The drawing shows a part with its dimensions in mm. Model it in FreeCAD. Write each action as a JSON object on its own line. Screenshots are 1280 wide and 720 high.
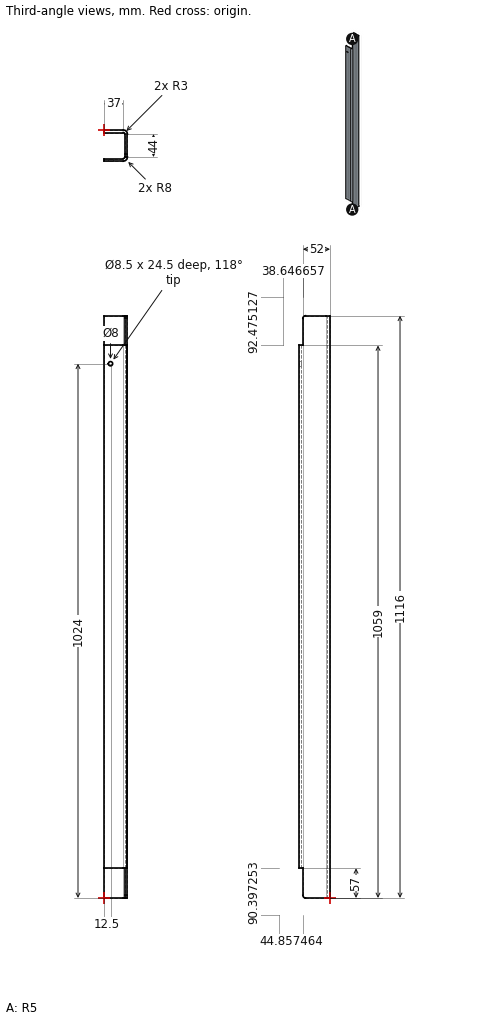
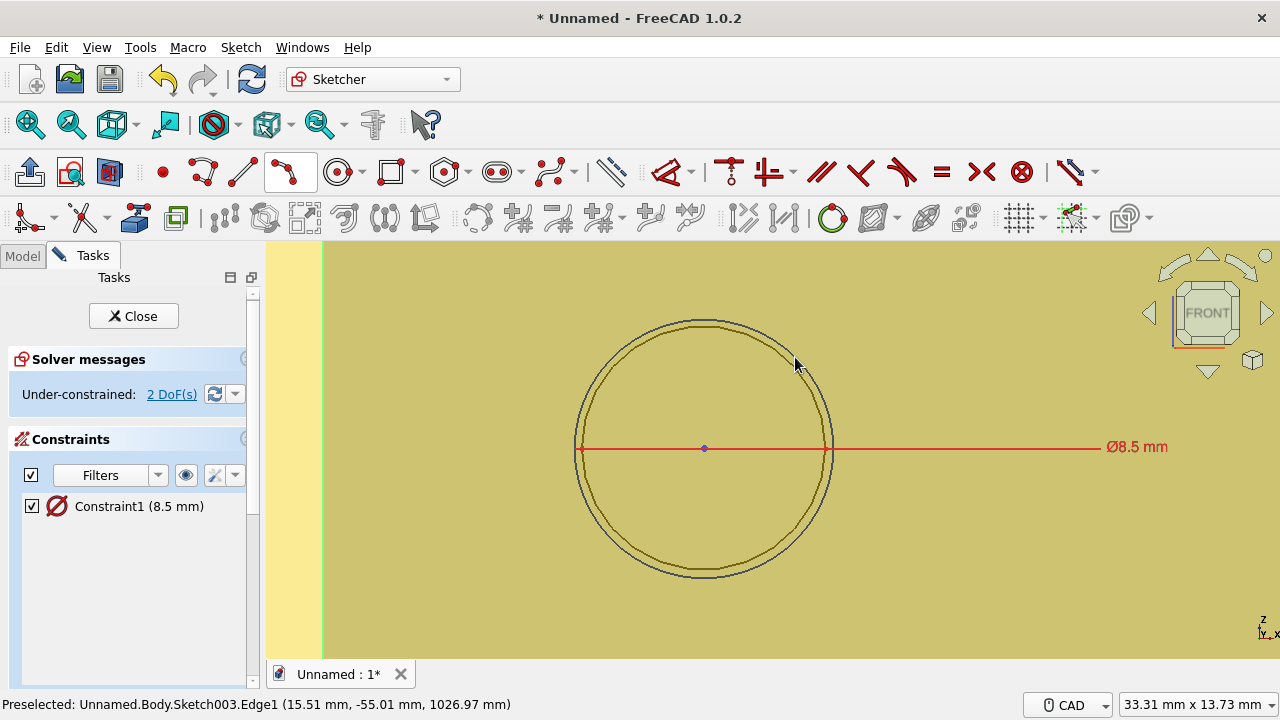
{"action": "key", "text": "d"}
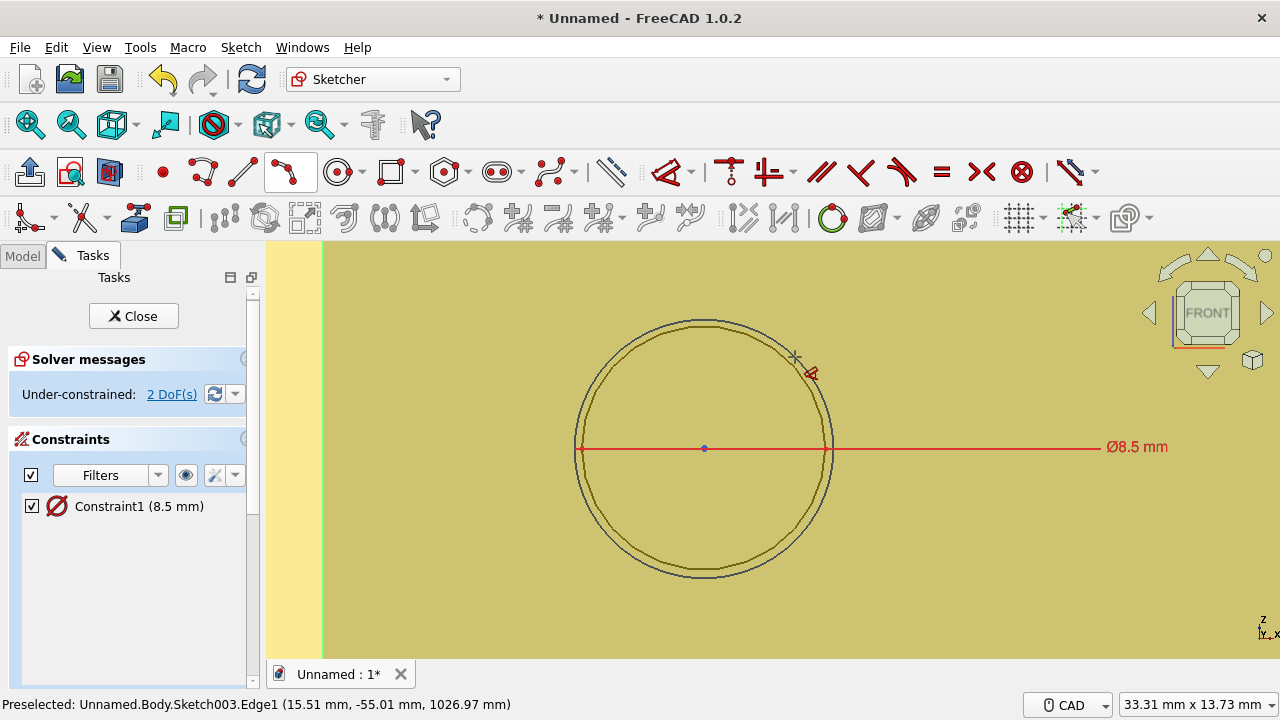
{"action": "left_click", "coordinate": [704, 449]}
{"action": "left_click", "coordinate": [514, 415]}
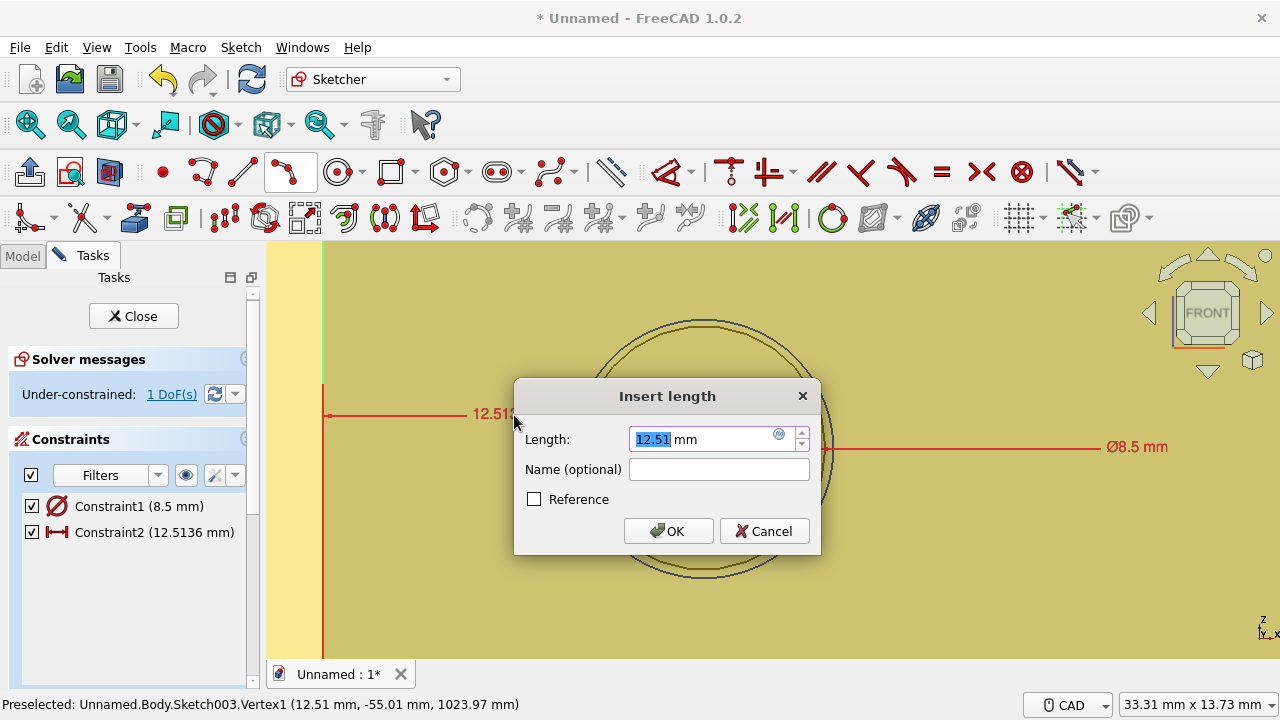
{"action": "type", "text": "12.5"}
{"action": "key", "text": "Return"}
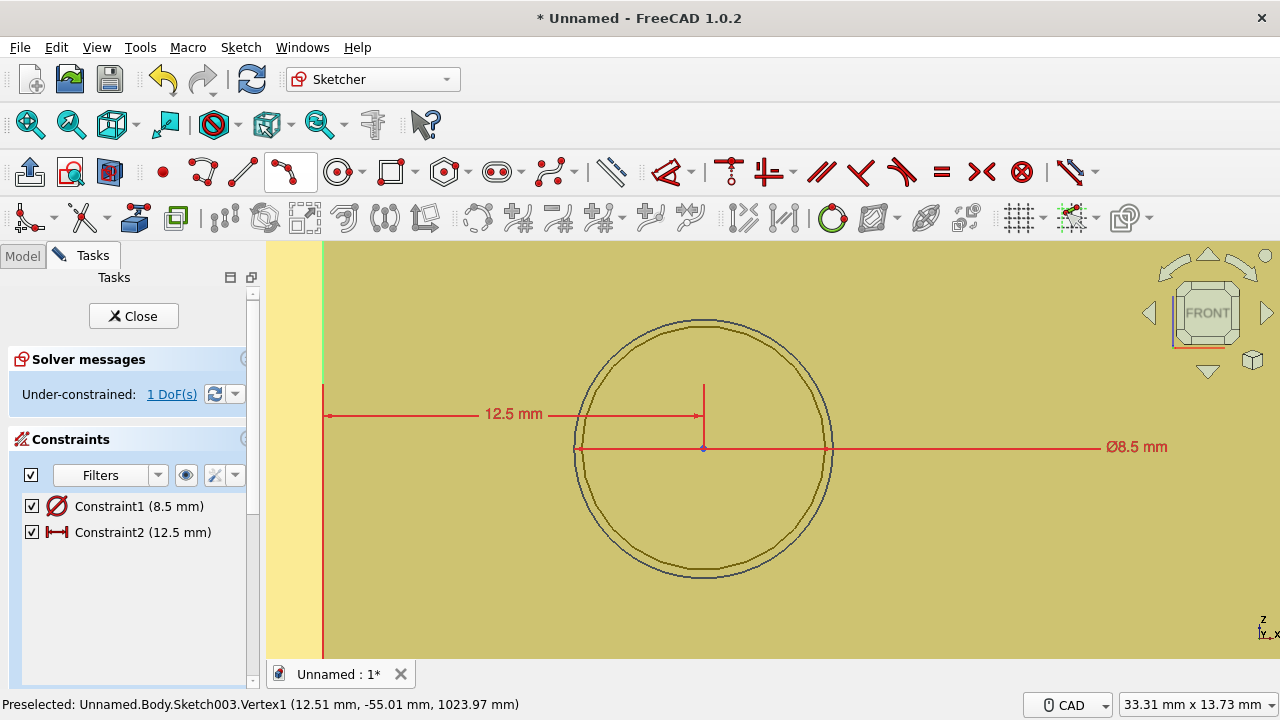
{"action": "left_click", "coordinate": [704, 449]}
{"action": "left_click", "coordinate": [738, 540]}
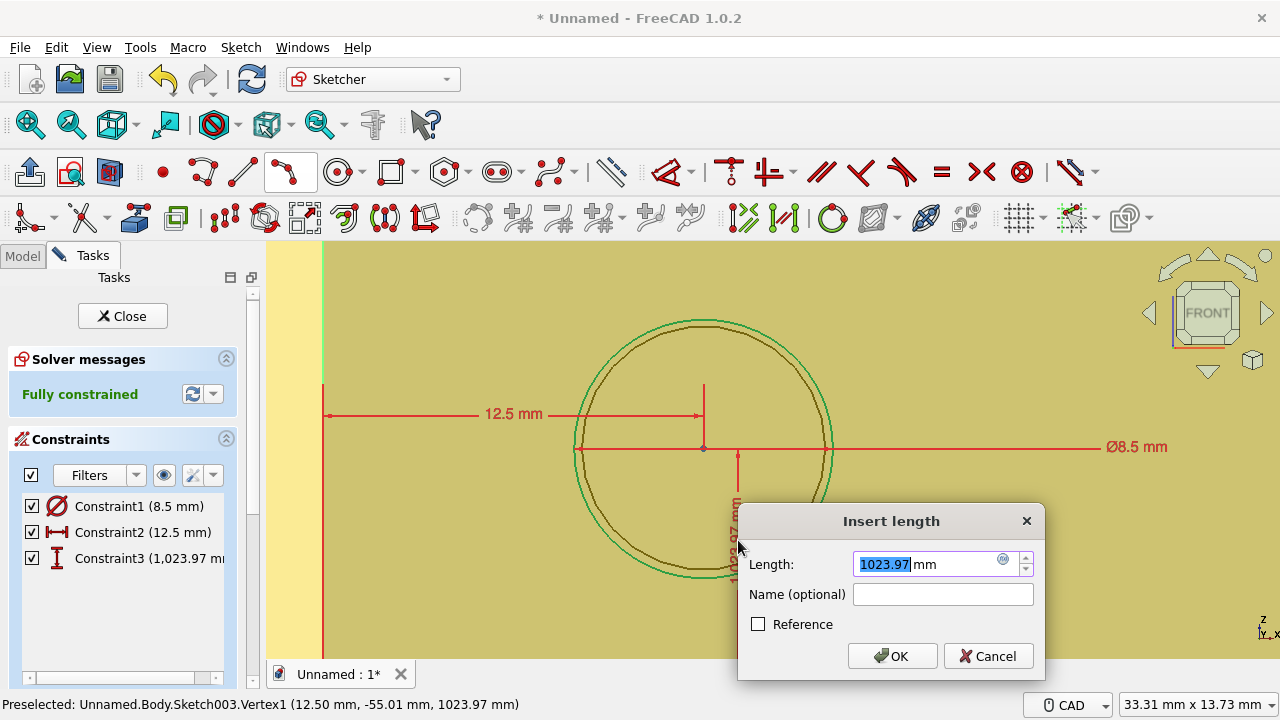
{"action": "type", "text": "1024"}
{"action": "key", "text": "Return"}
{"action": "key", "text": "Escape"}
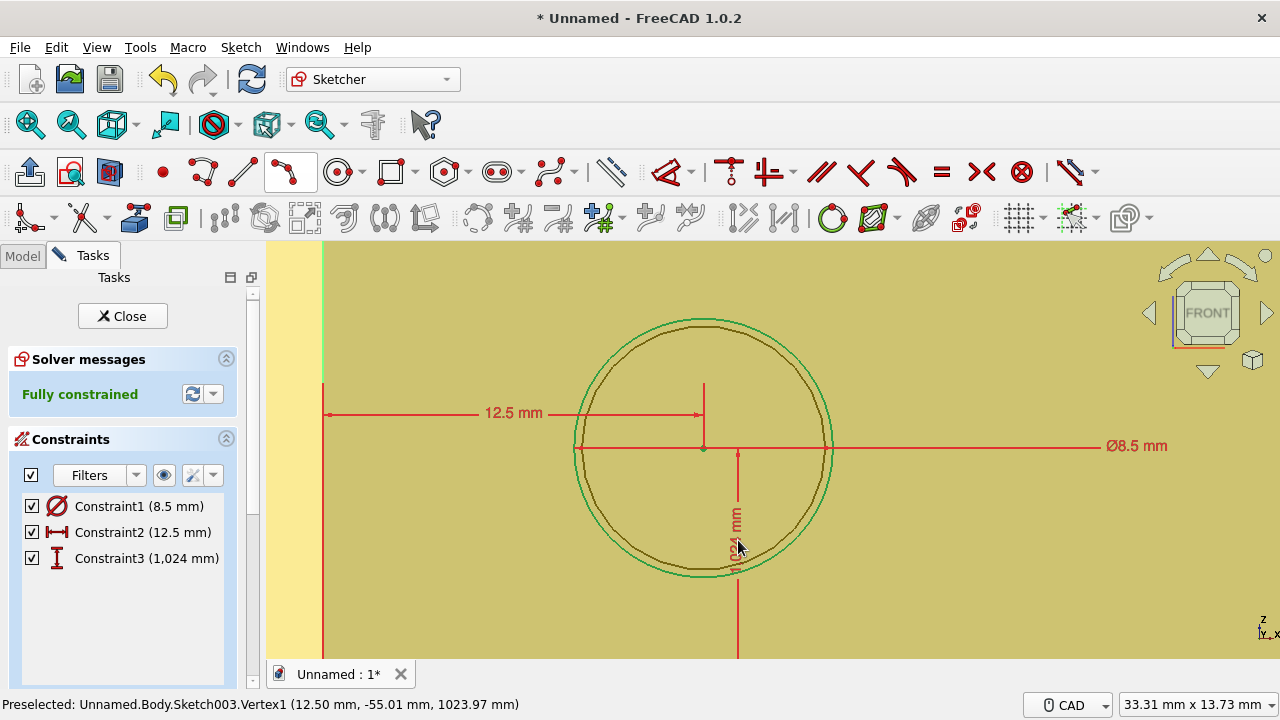
{"action": "left_click", "coordinate": [123, 316]}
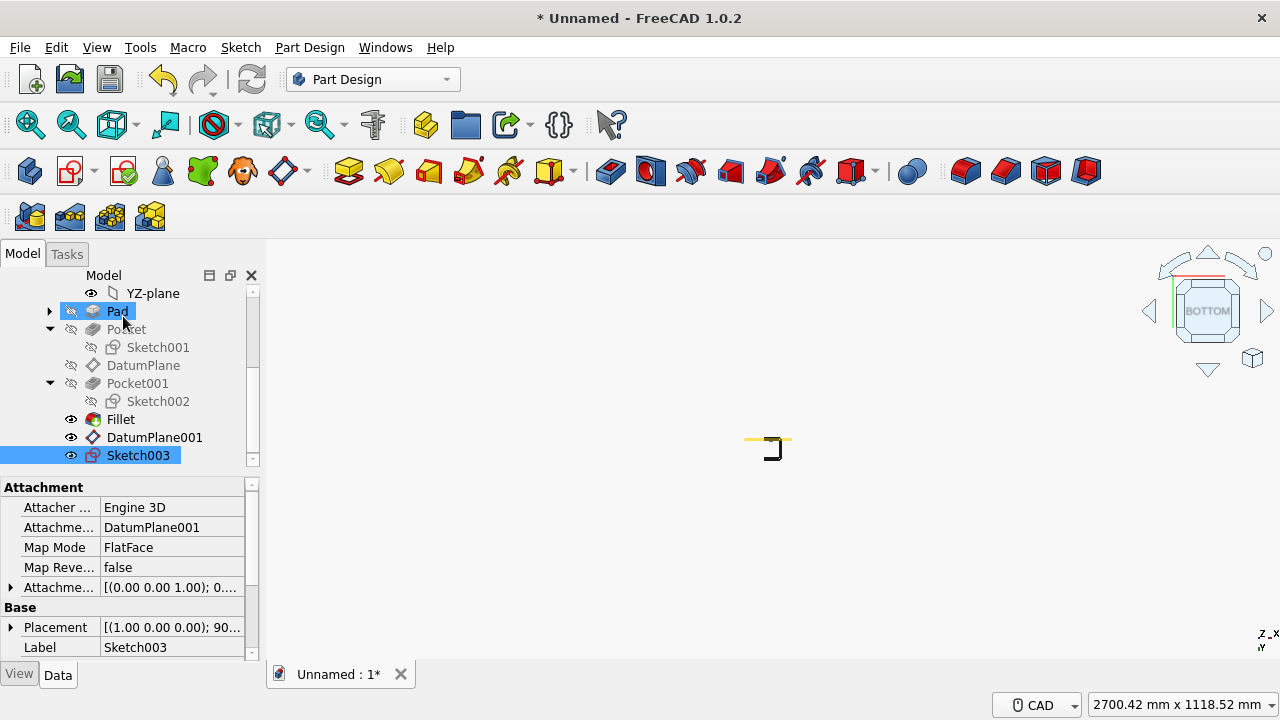
{"action": "left_click", "coordinate": [652, 172]}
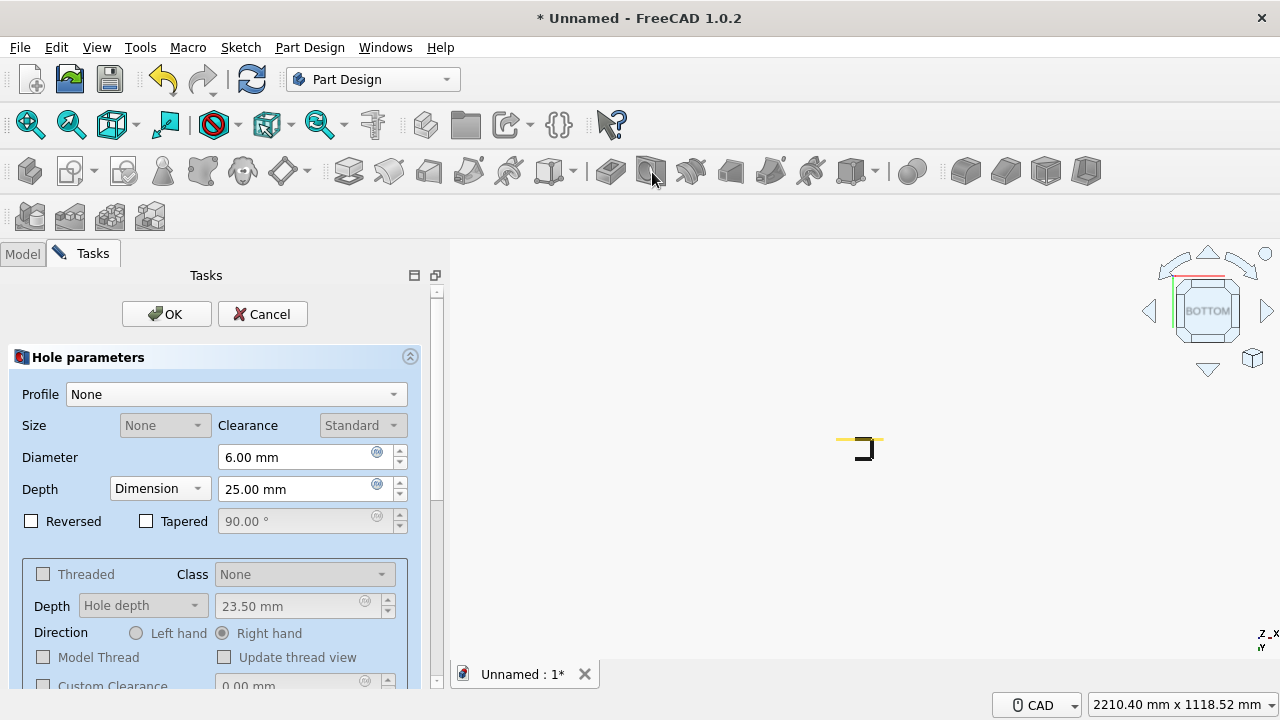
{"action": "triple_click", "coordinate": [305, 457]}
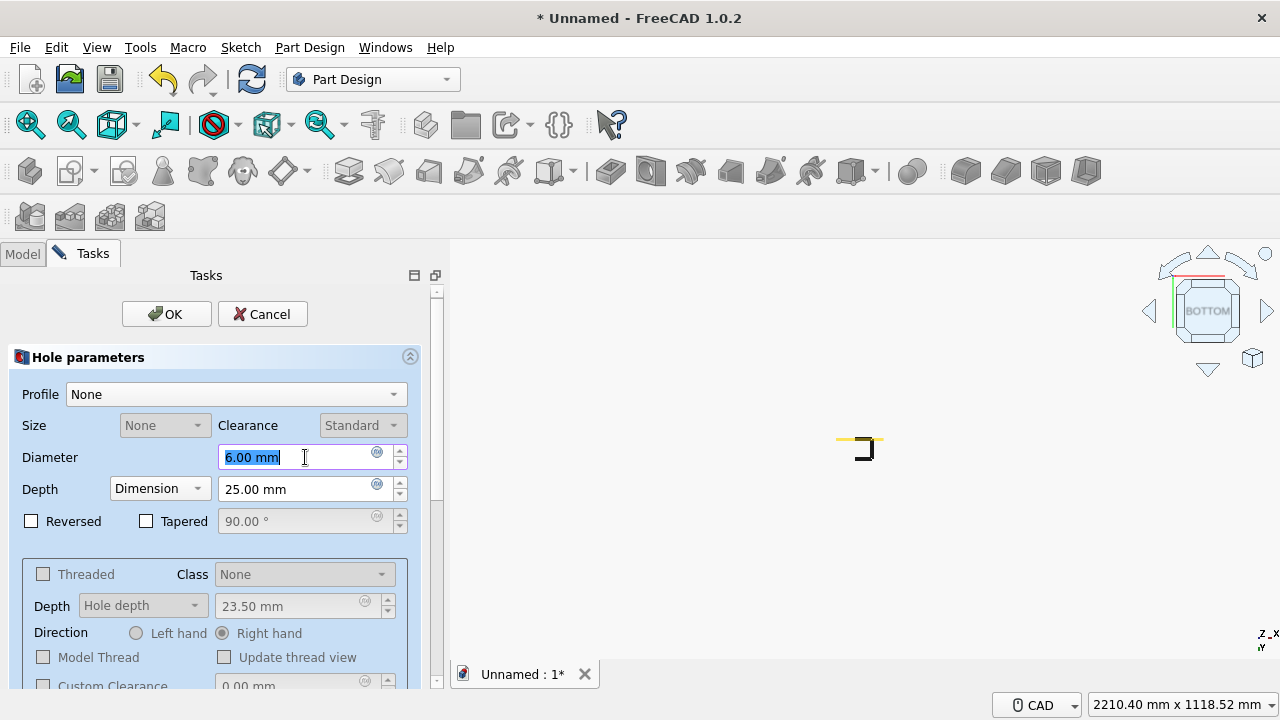
{"action": "type", "text": "8.5"}
{"action": "key", "text": "Tab"}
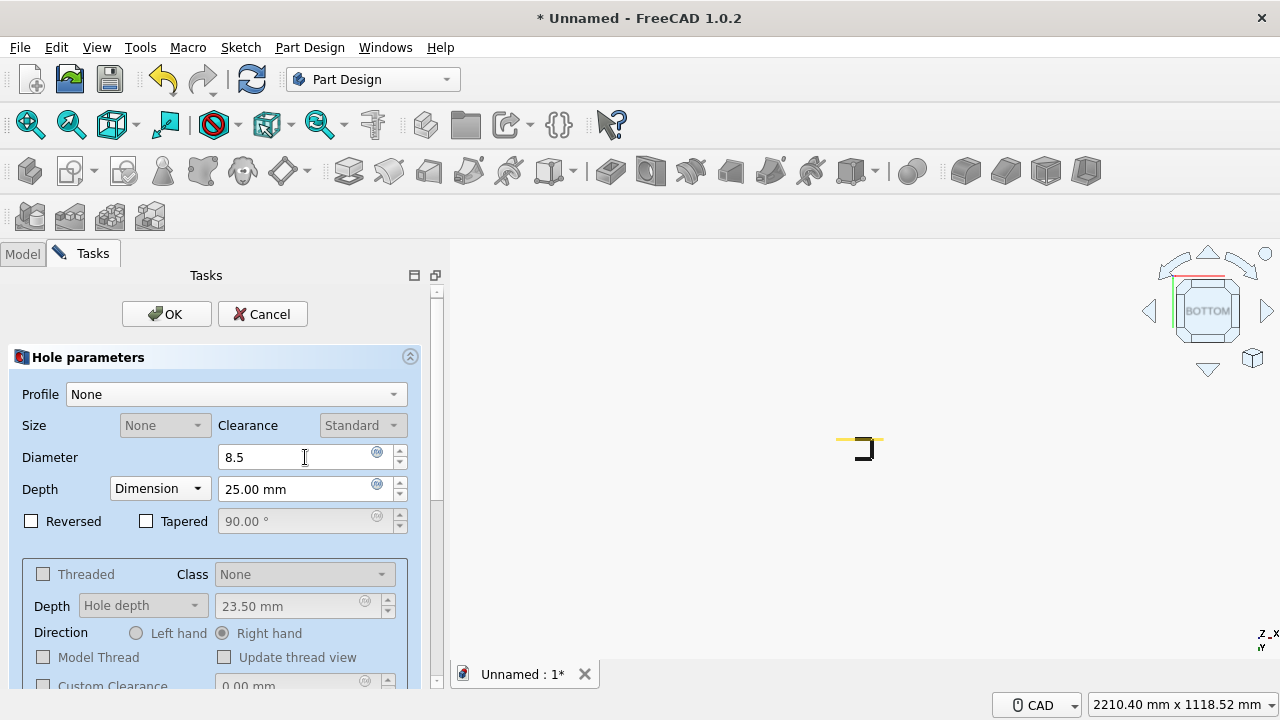
{"action": "triple_click", "coordinate": [305, 489]}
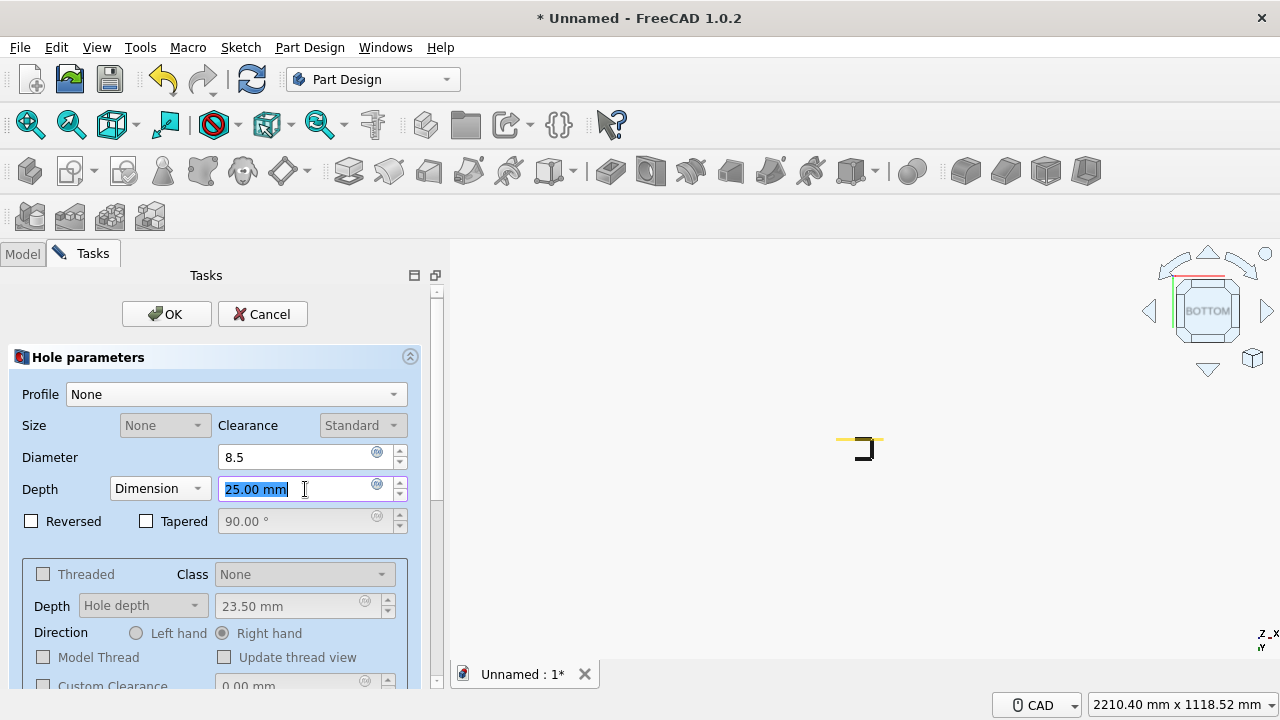
{"action": "type", "text": "24.5"}
{"action": "key", "text": "Tab"}